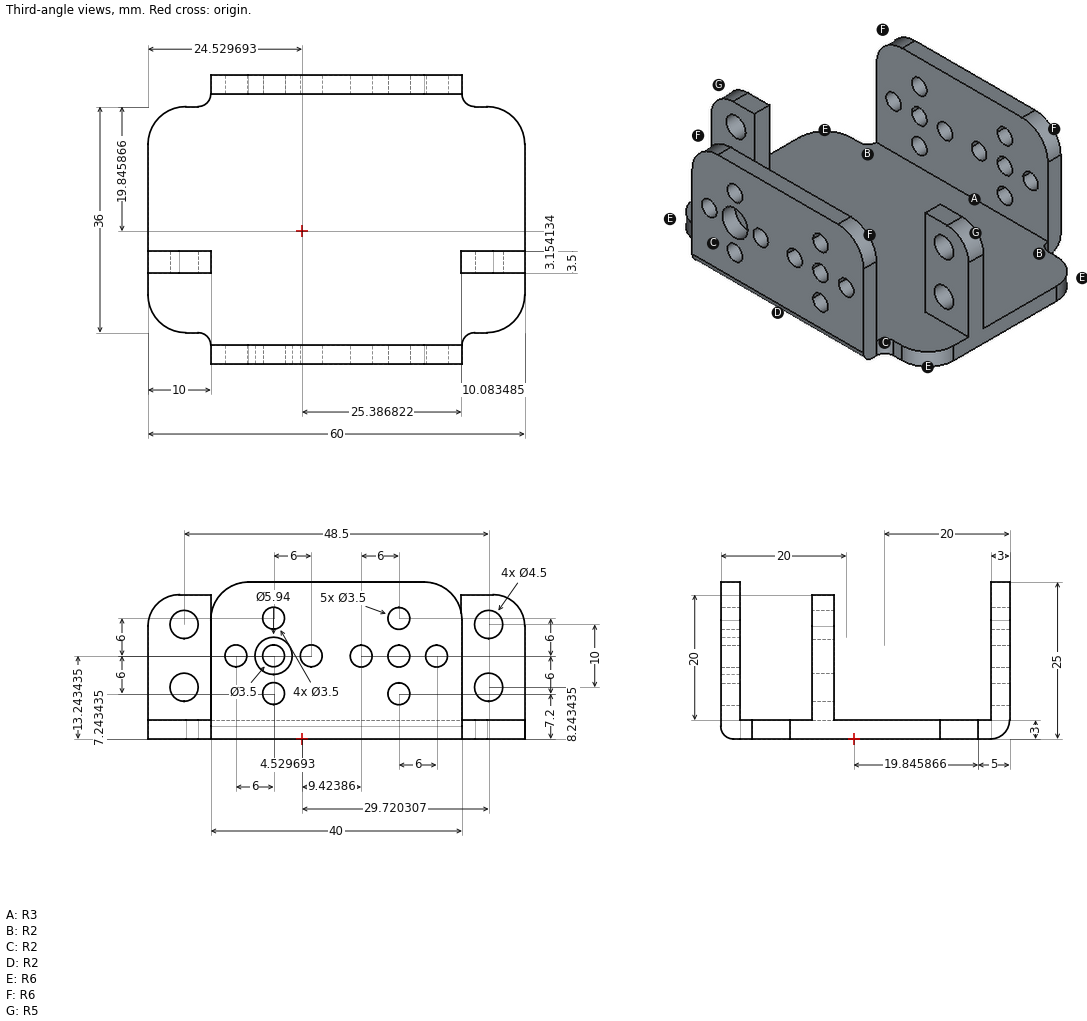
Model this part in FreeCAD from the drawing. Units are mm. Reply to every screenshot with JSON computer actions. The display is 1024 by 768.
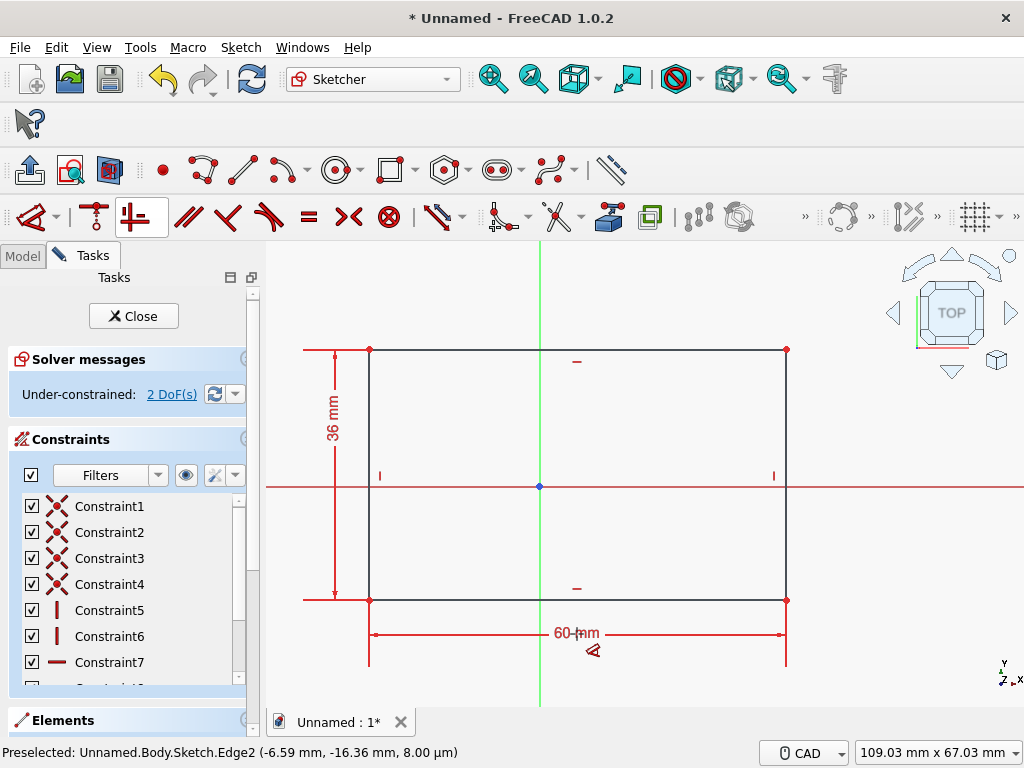
{"action": "left_click", "coordinate": [369, 350]}
{"action": "left_click", "coordinate": [454, 316]}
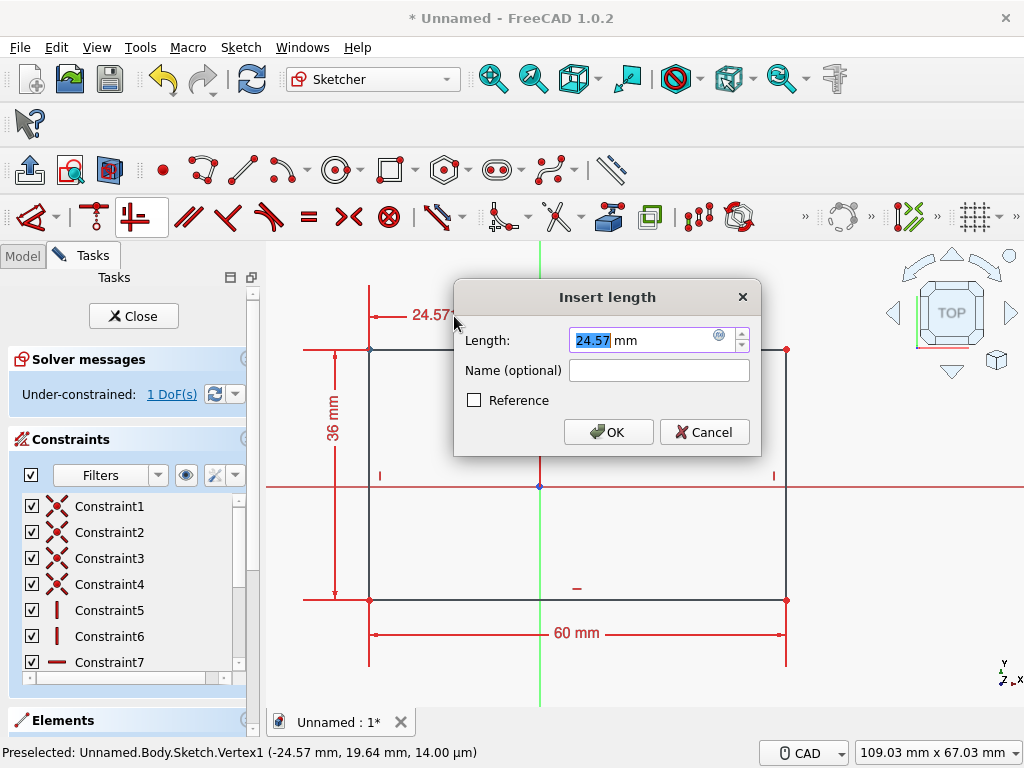
{"action": "type", "text": "24.529693"}
{"action": "key", "text": "Return"}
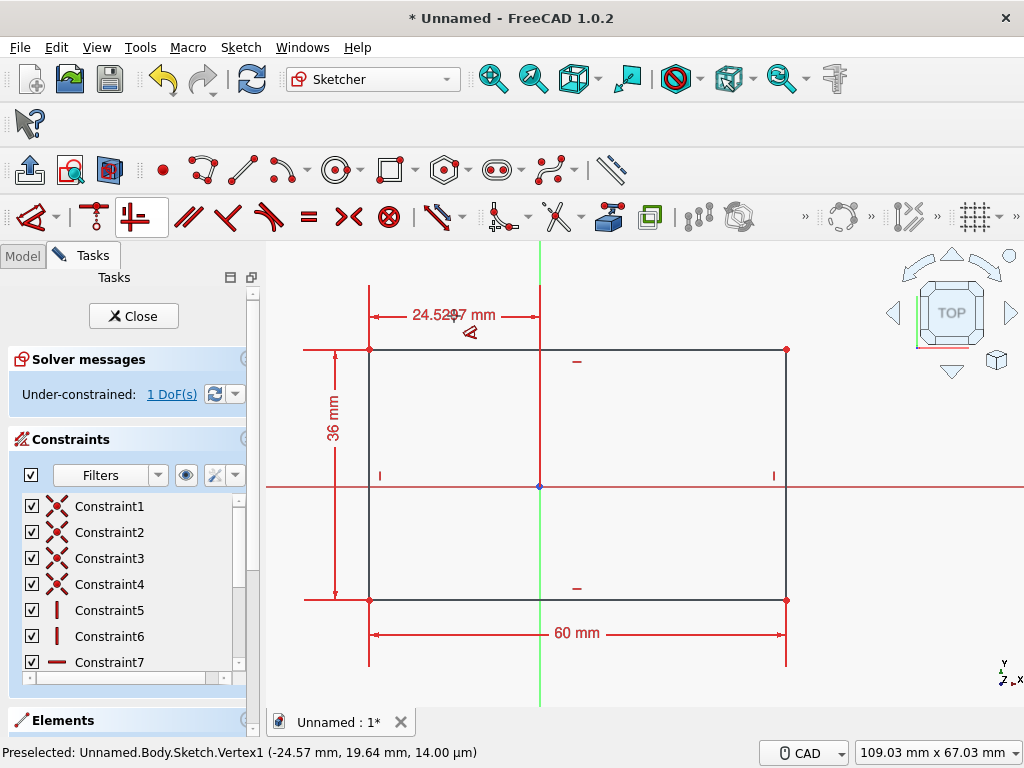
{"action": "left_click", "coordinate": [369, 350]}
{"action": "left_click", "coordinate": [335, 387]}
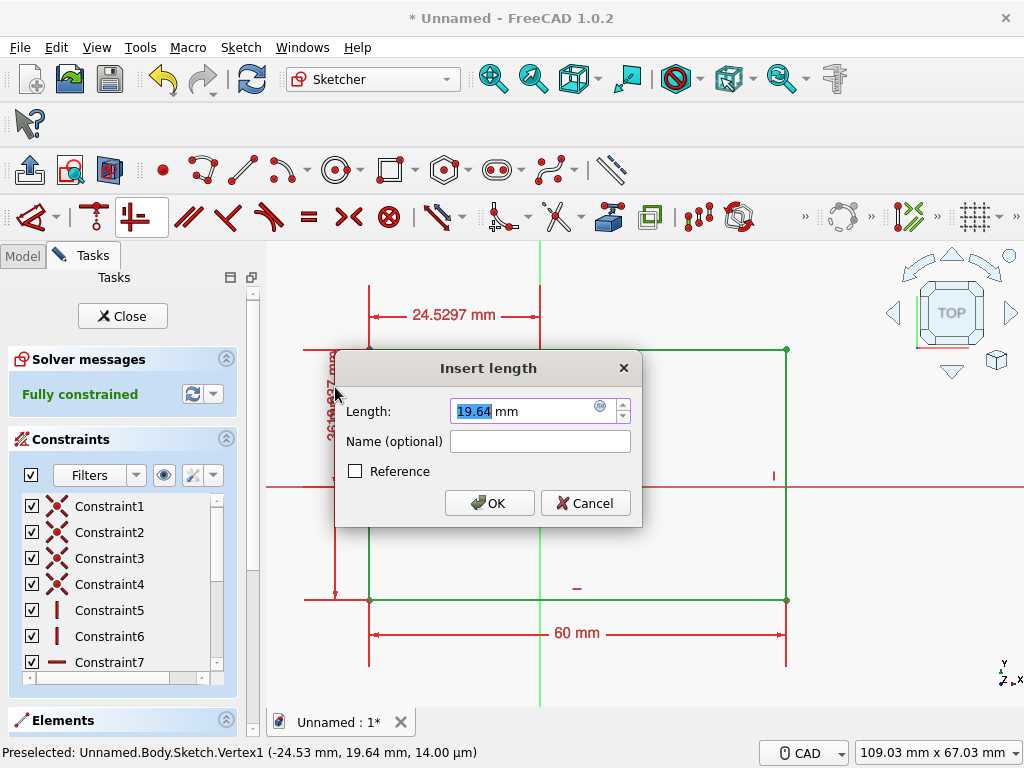
{"action": "type", "text": "19.845866"}
{"action": "key", "text": "Return"}
{"action": "key", "text": "Escape"}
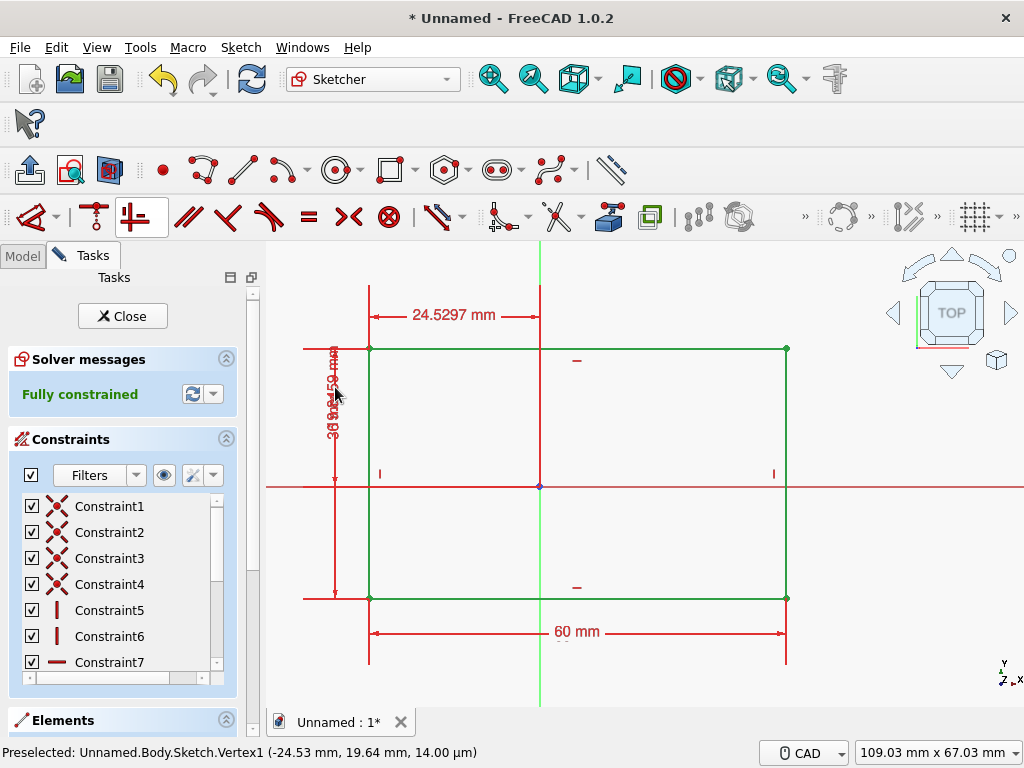
{"action": "left_click", "coordinate": [123, 316]}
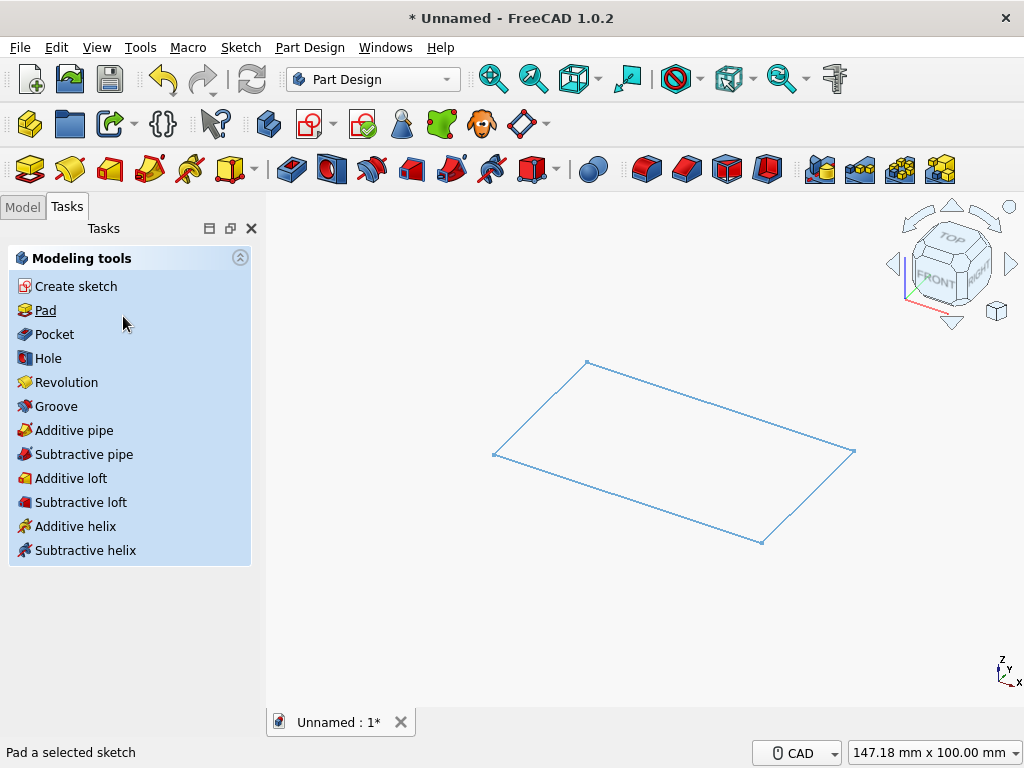
{"action": "left_click", "coordinate": [30, 170]}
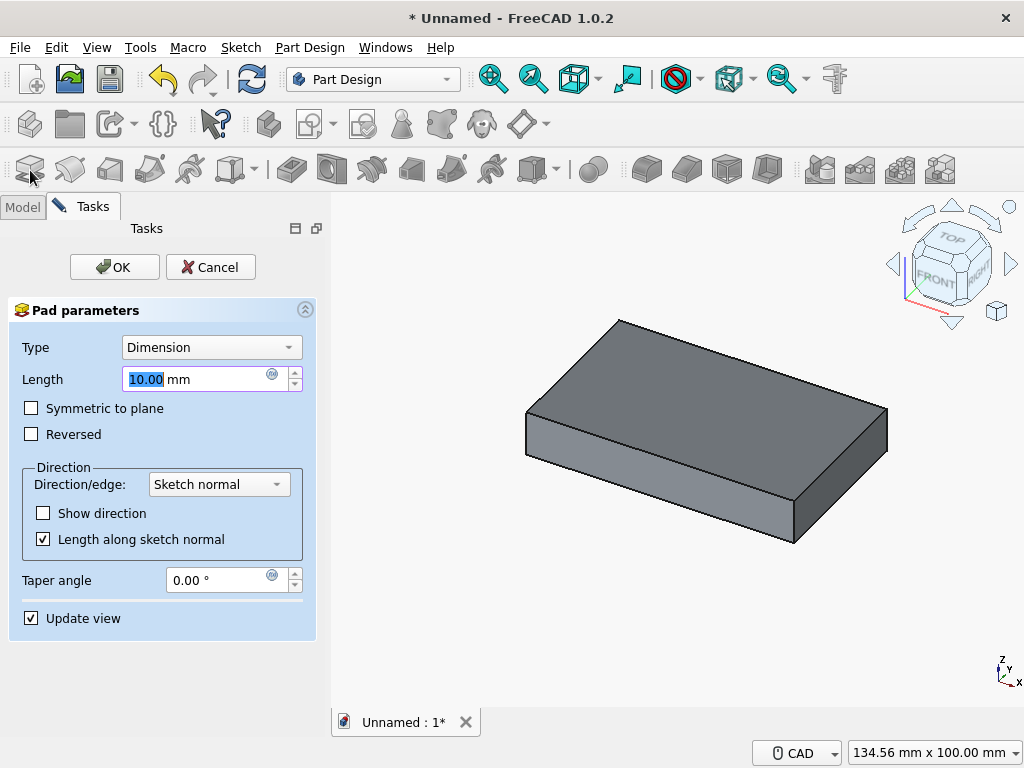
{"action": "type", "text": "3"}
{"action": "key", "text": "Tab"}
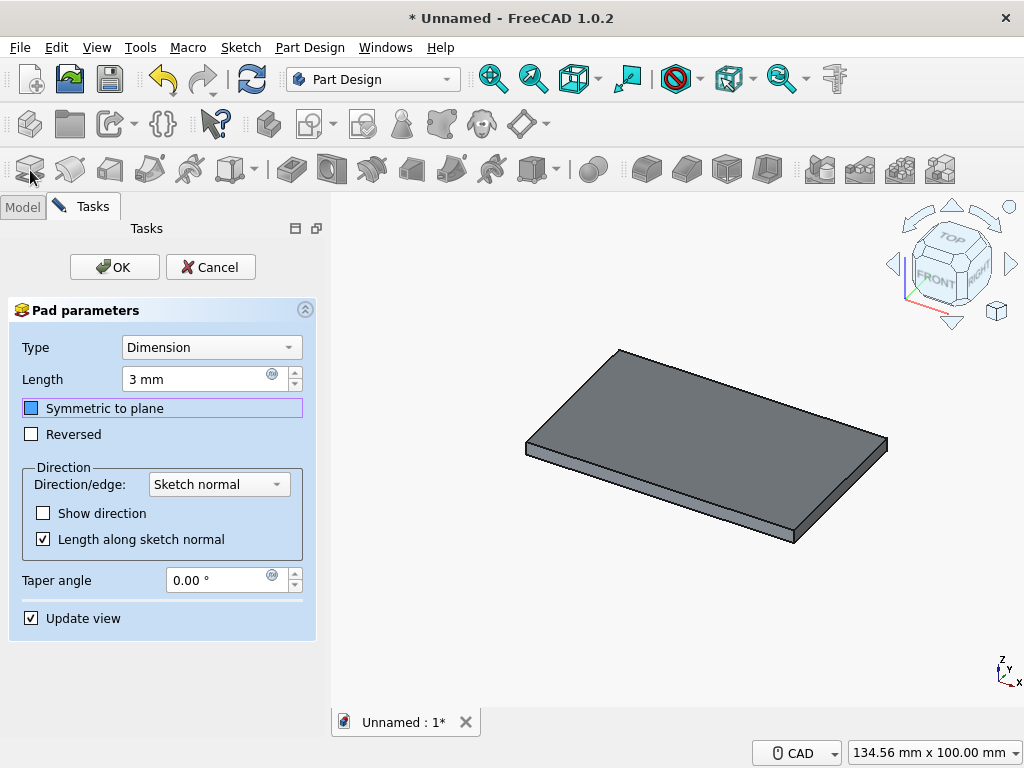
{"action": "left_click", "coordinate": [115, 267]}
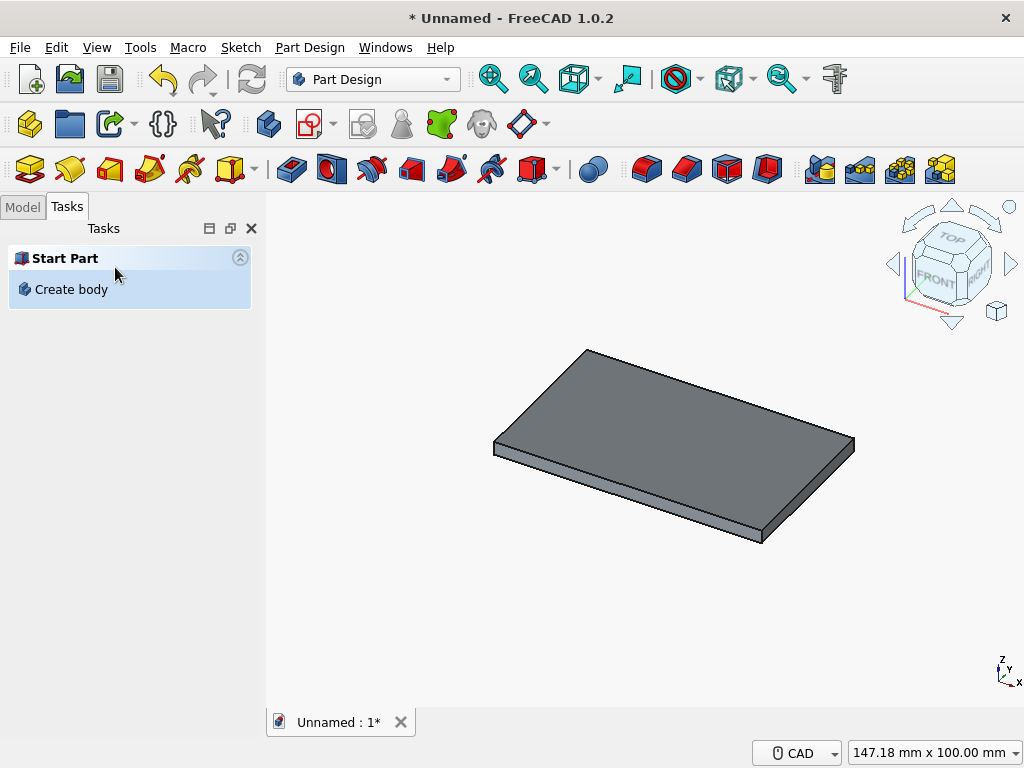
{"action": "left_click", "coordinate": [23, 206]}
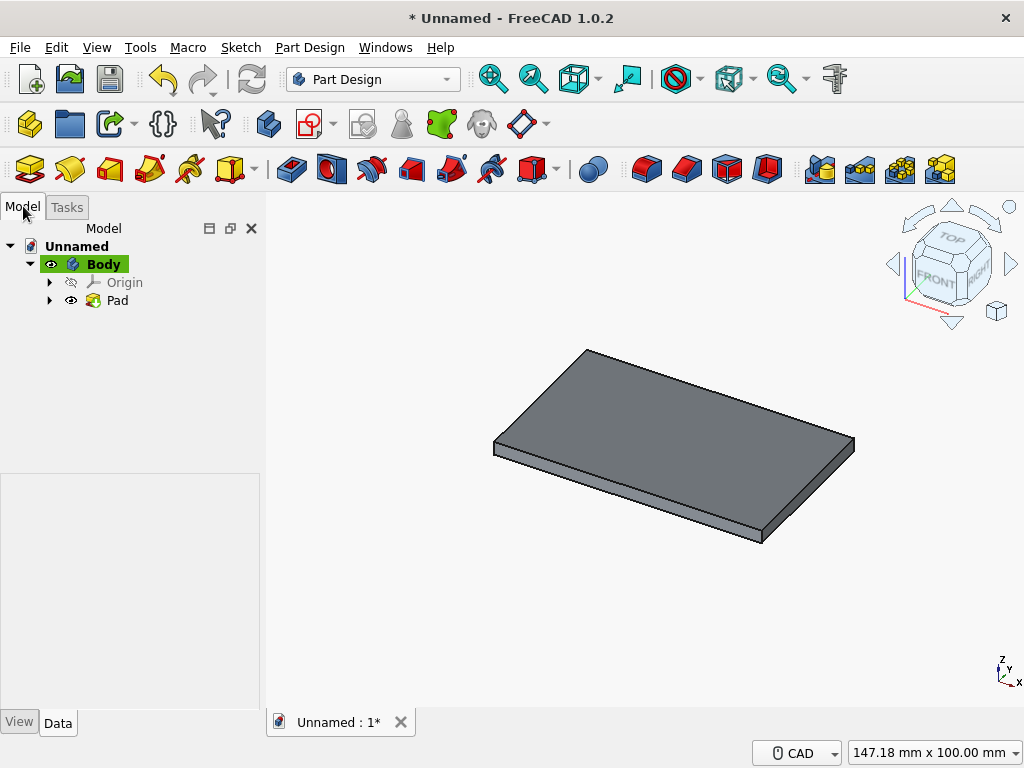
{"action": "left_click", "coordinate": [50, 282]}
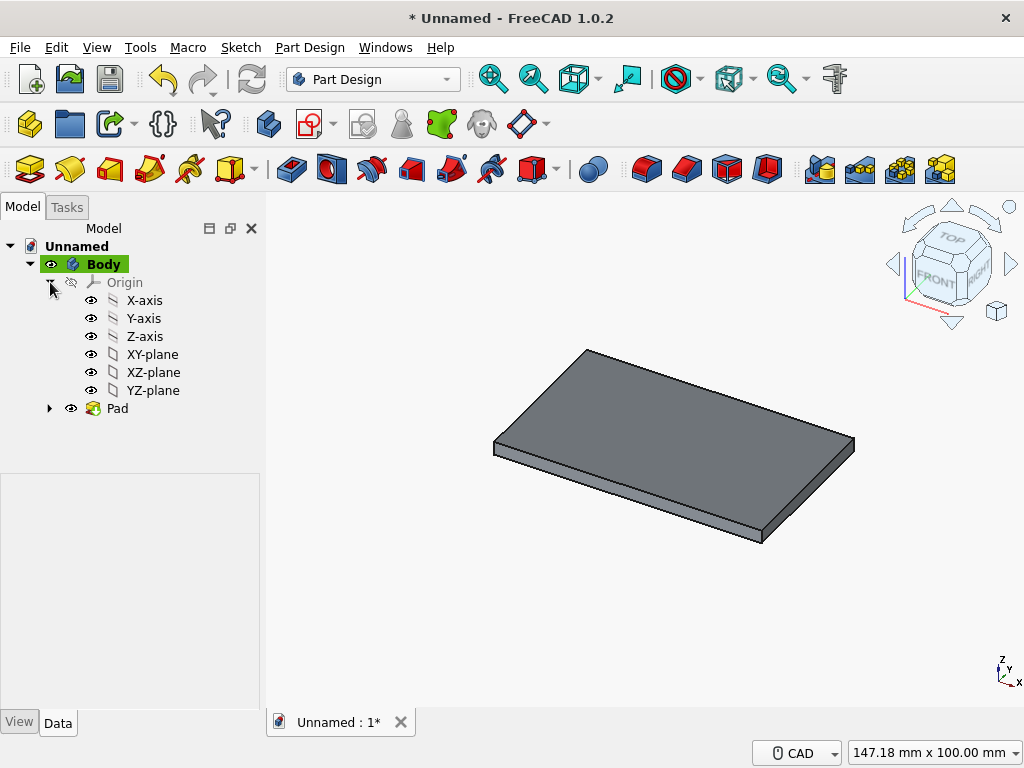
{"action": "left_click", "coordinate": [136, 390]}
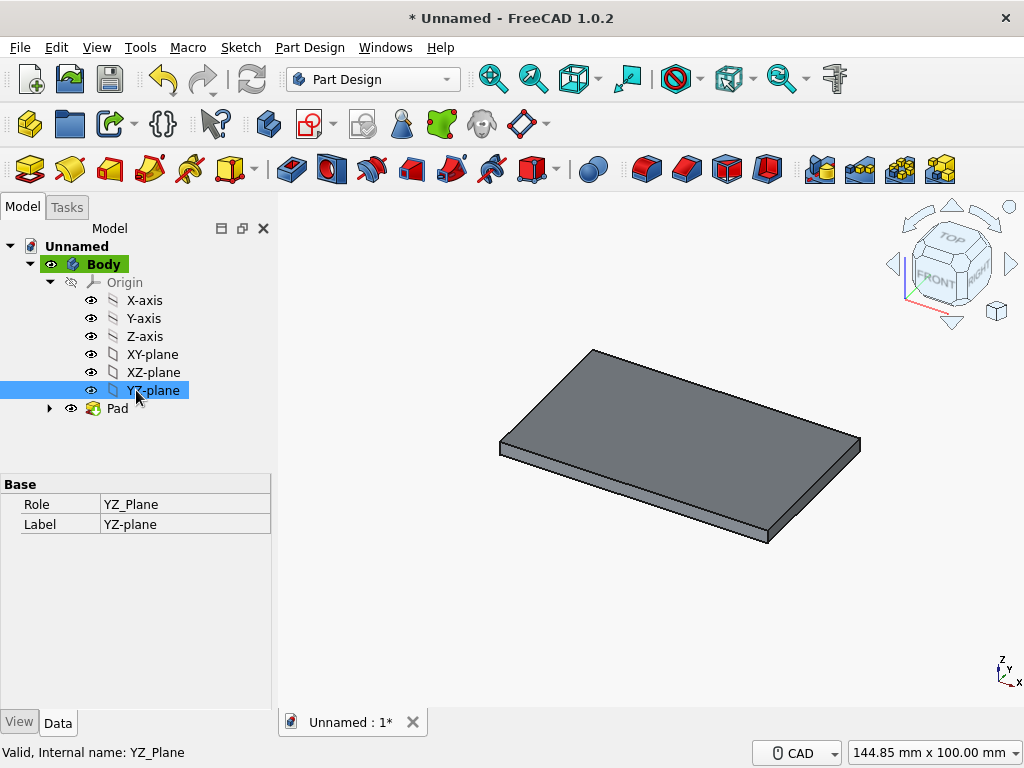
{"action": "left_click", "coordinate": [522, 124]}